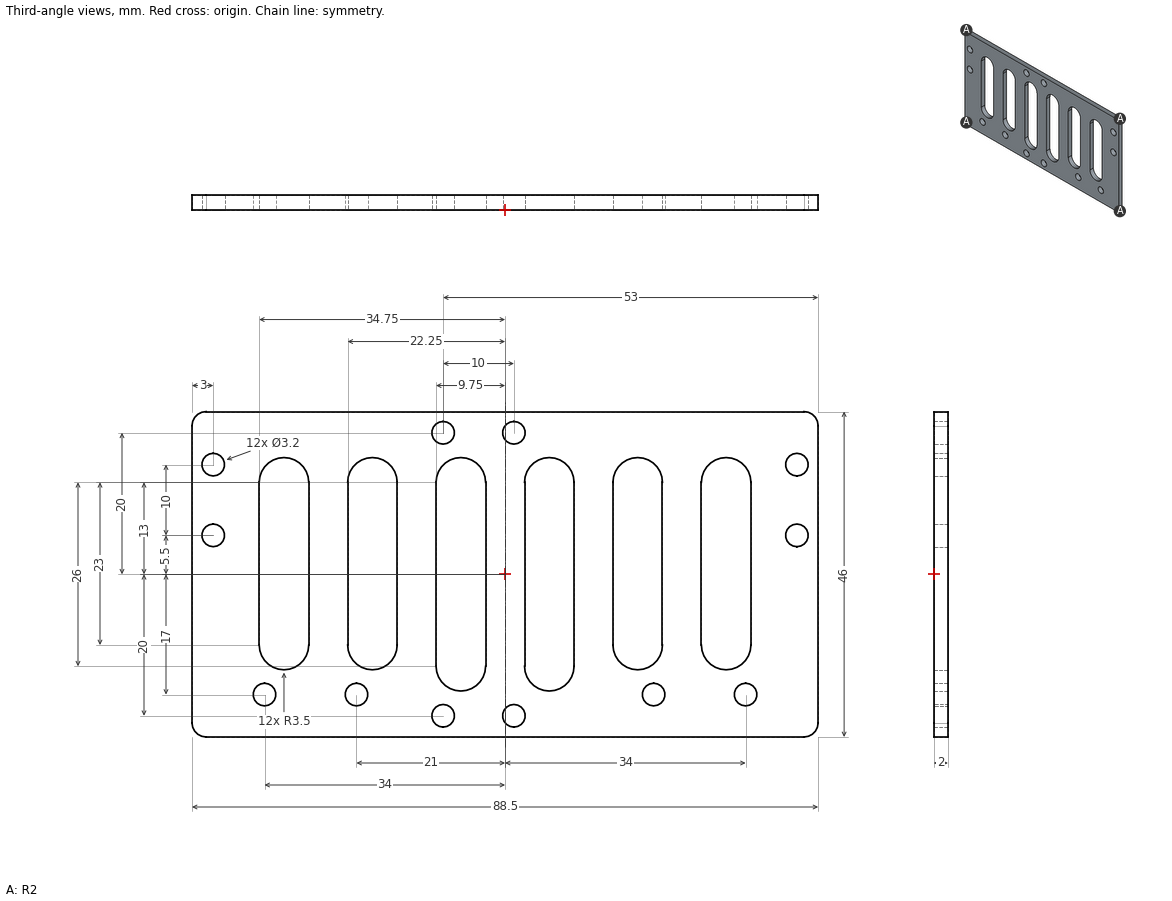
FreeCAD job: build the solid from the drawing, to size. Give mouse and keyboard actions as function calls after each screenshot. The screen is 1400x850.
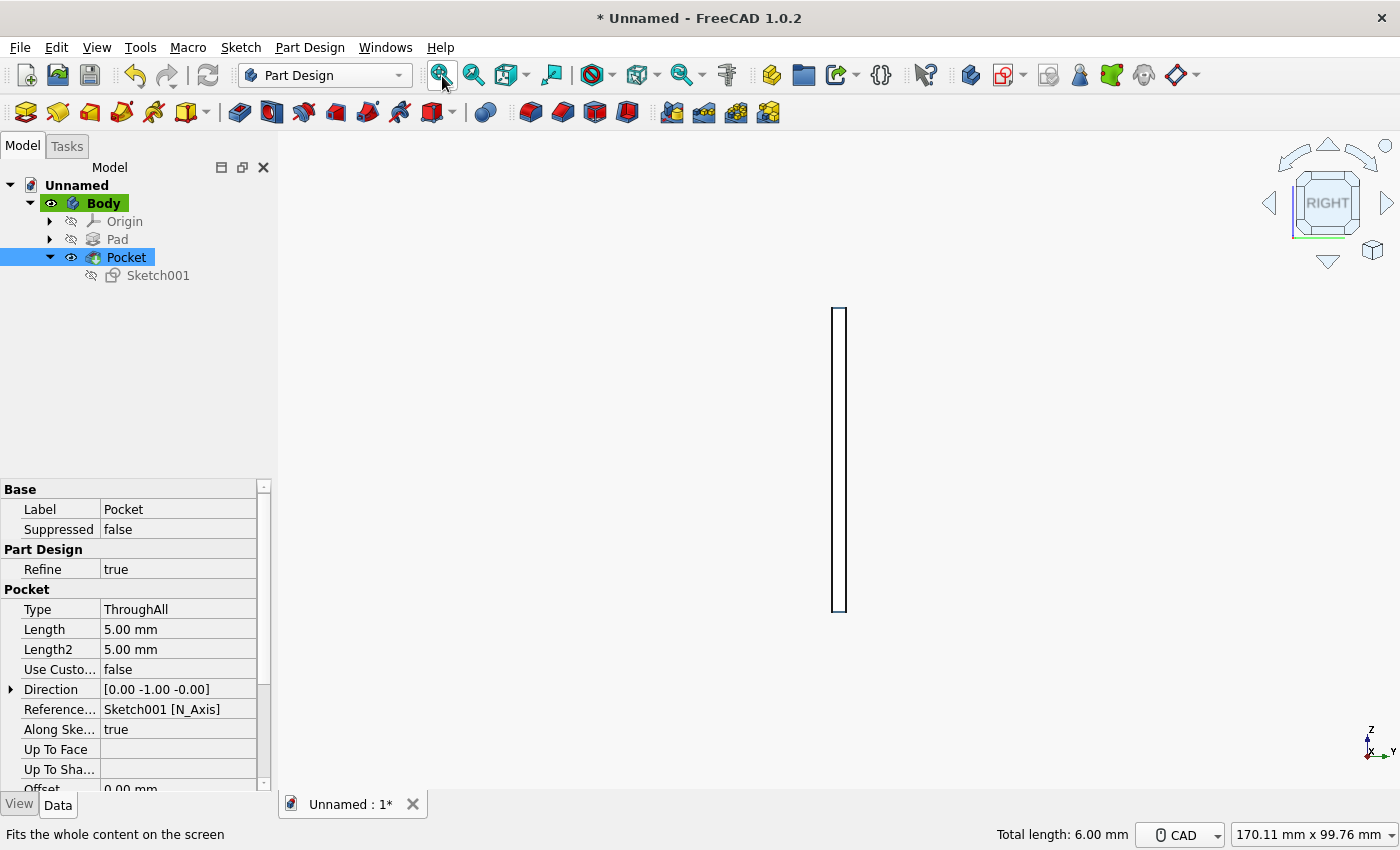
key(5)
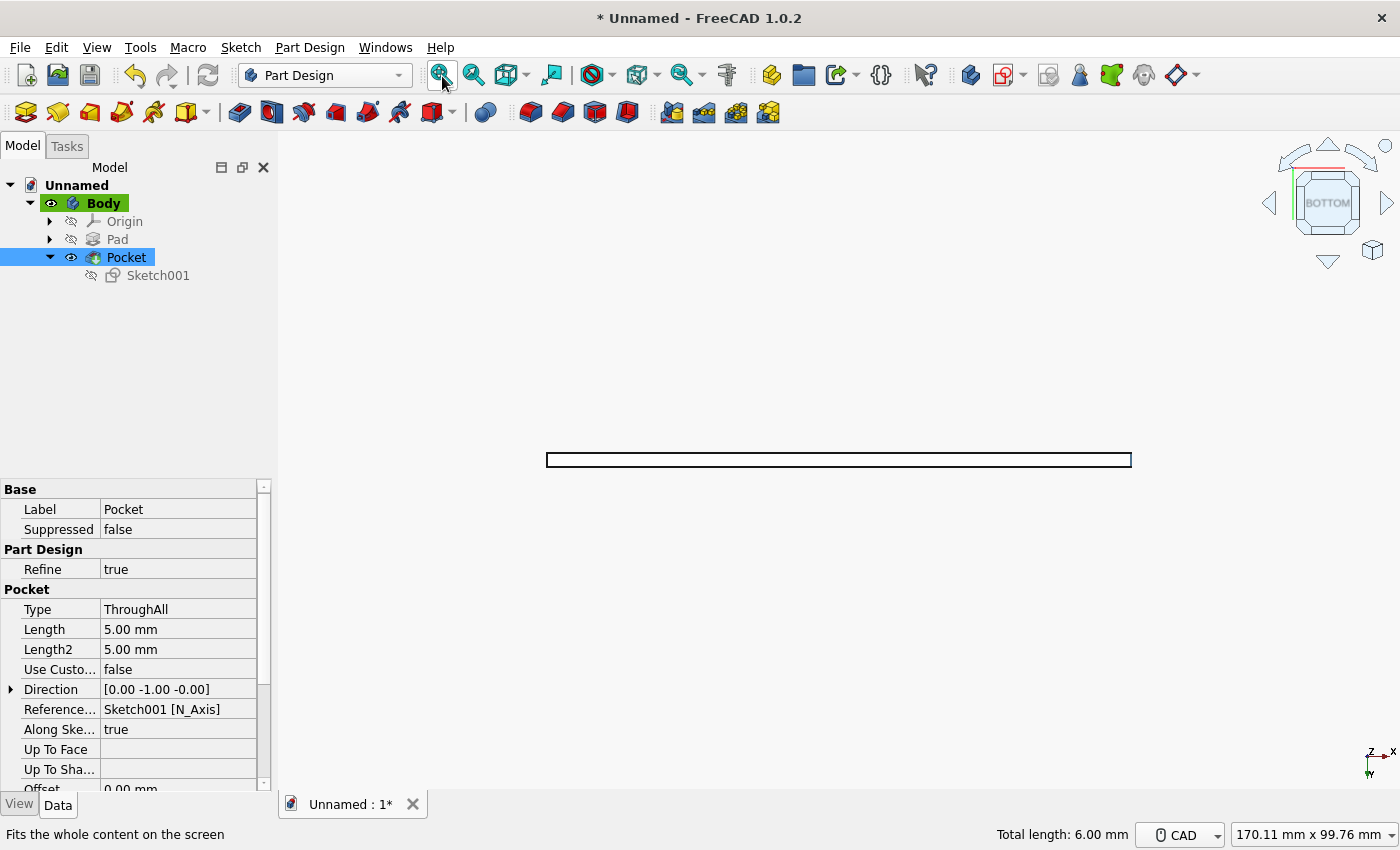
click(547, 459, ctrl)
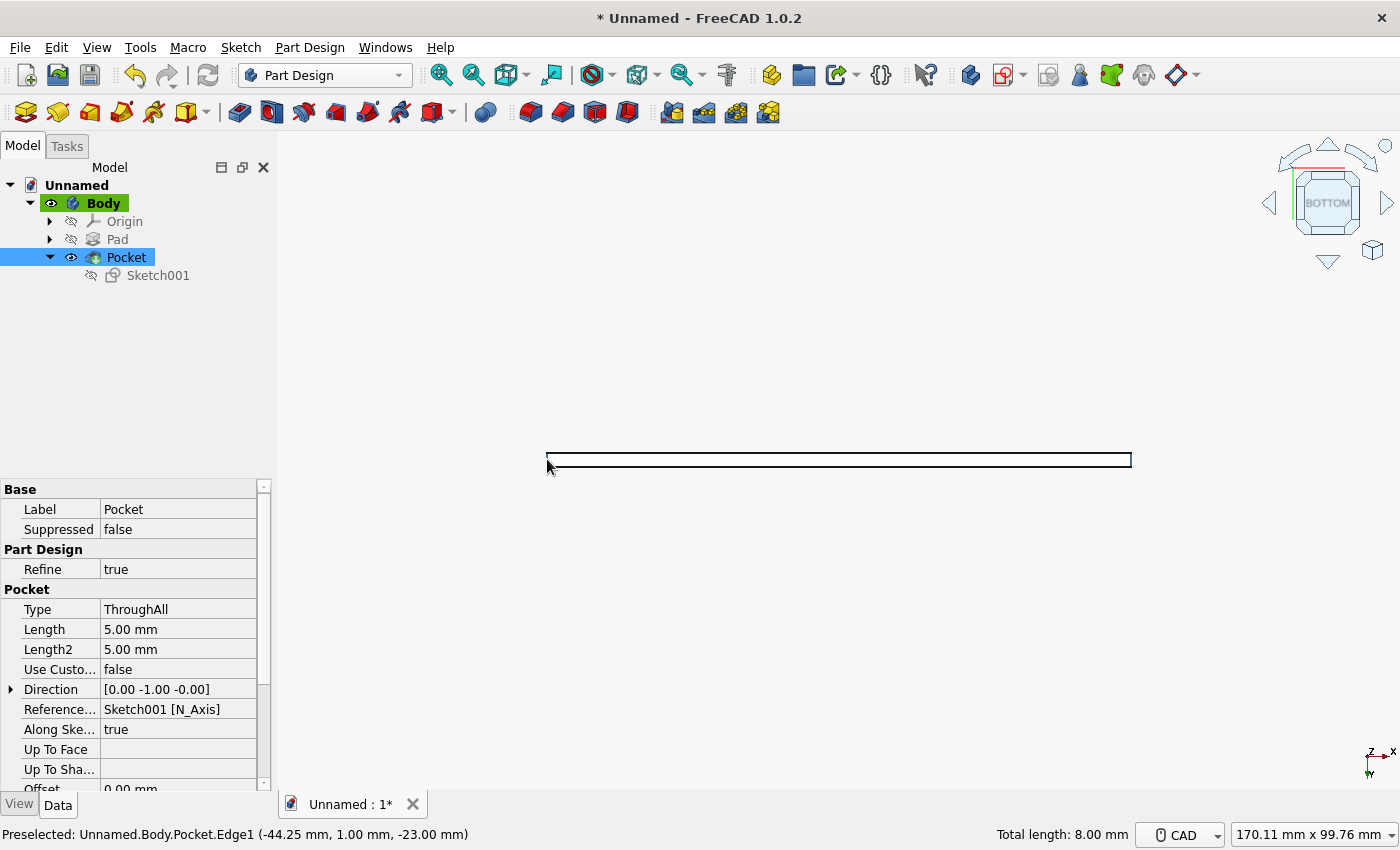
click(532, 112)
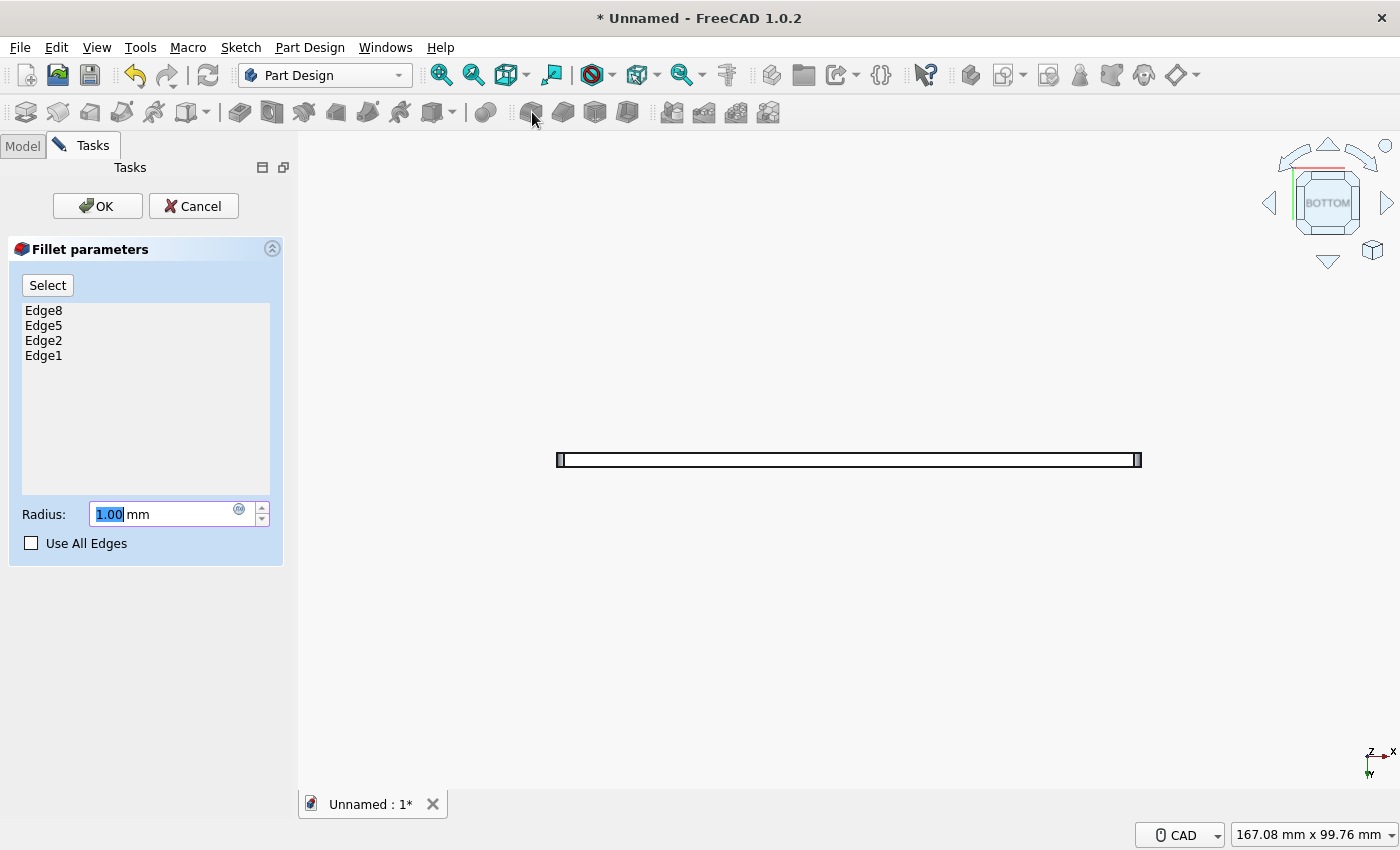
text(2)
key(Tab)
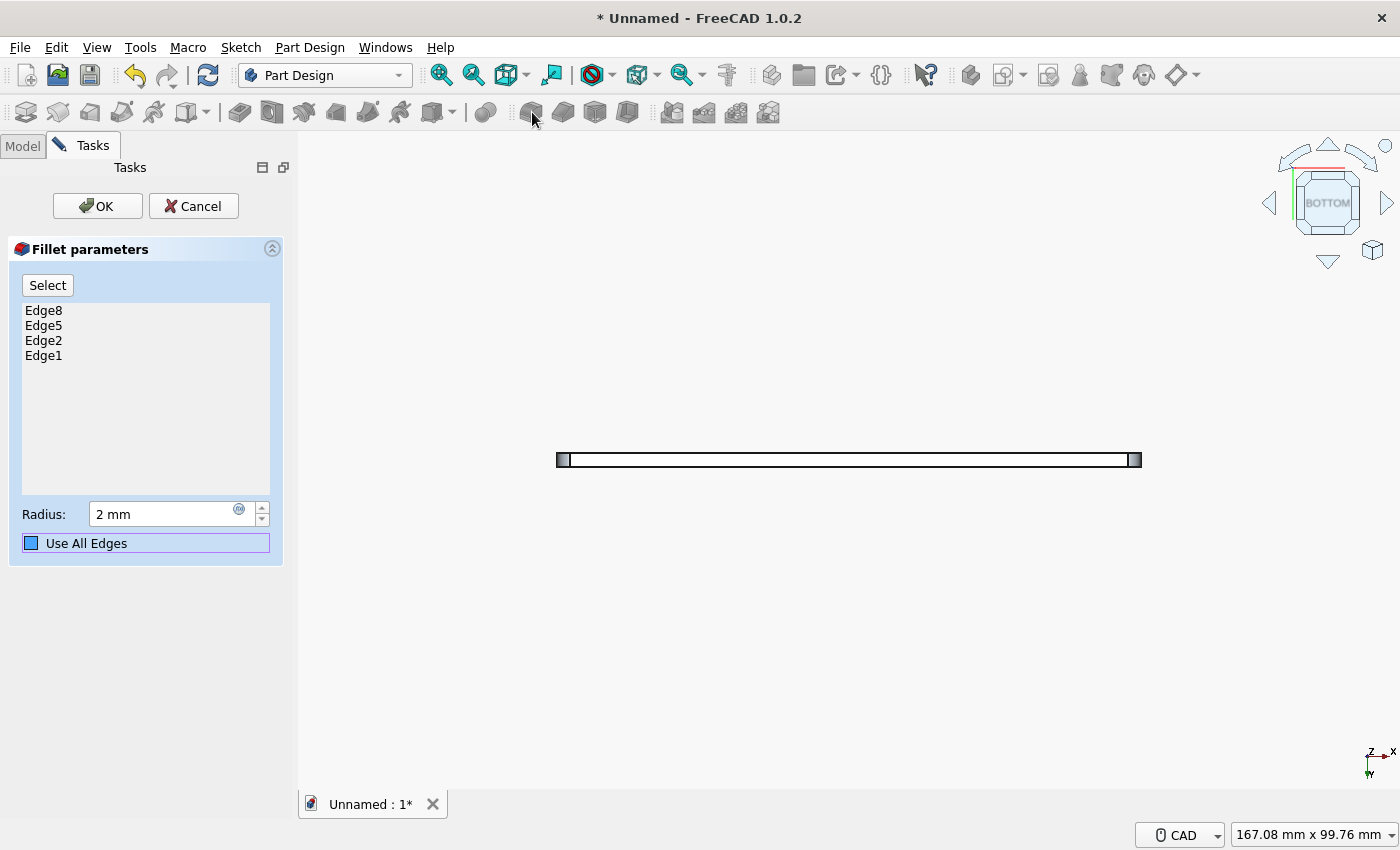
click(98, 206)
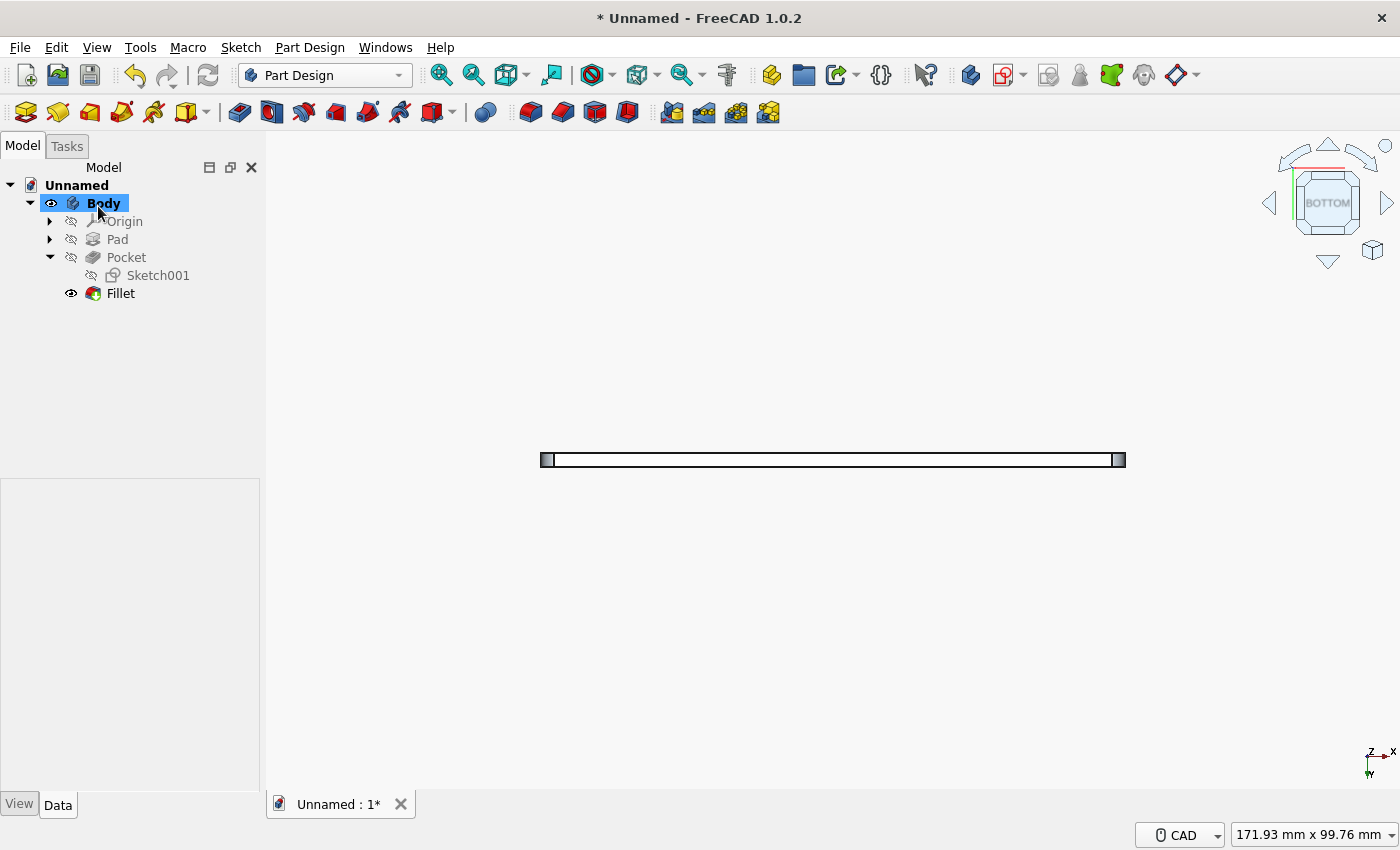
key(0)